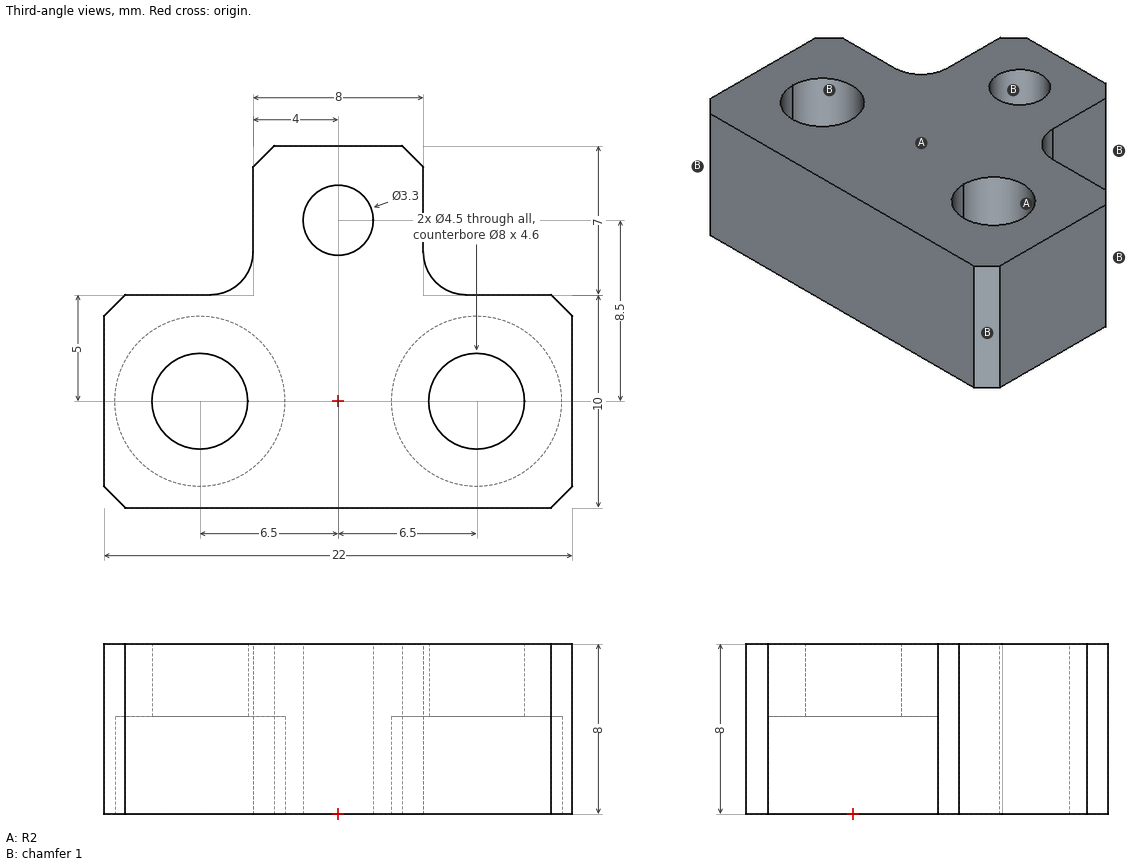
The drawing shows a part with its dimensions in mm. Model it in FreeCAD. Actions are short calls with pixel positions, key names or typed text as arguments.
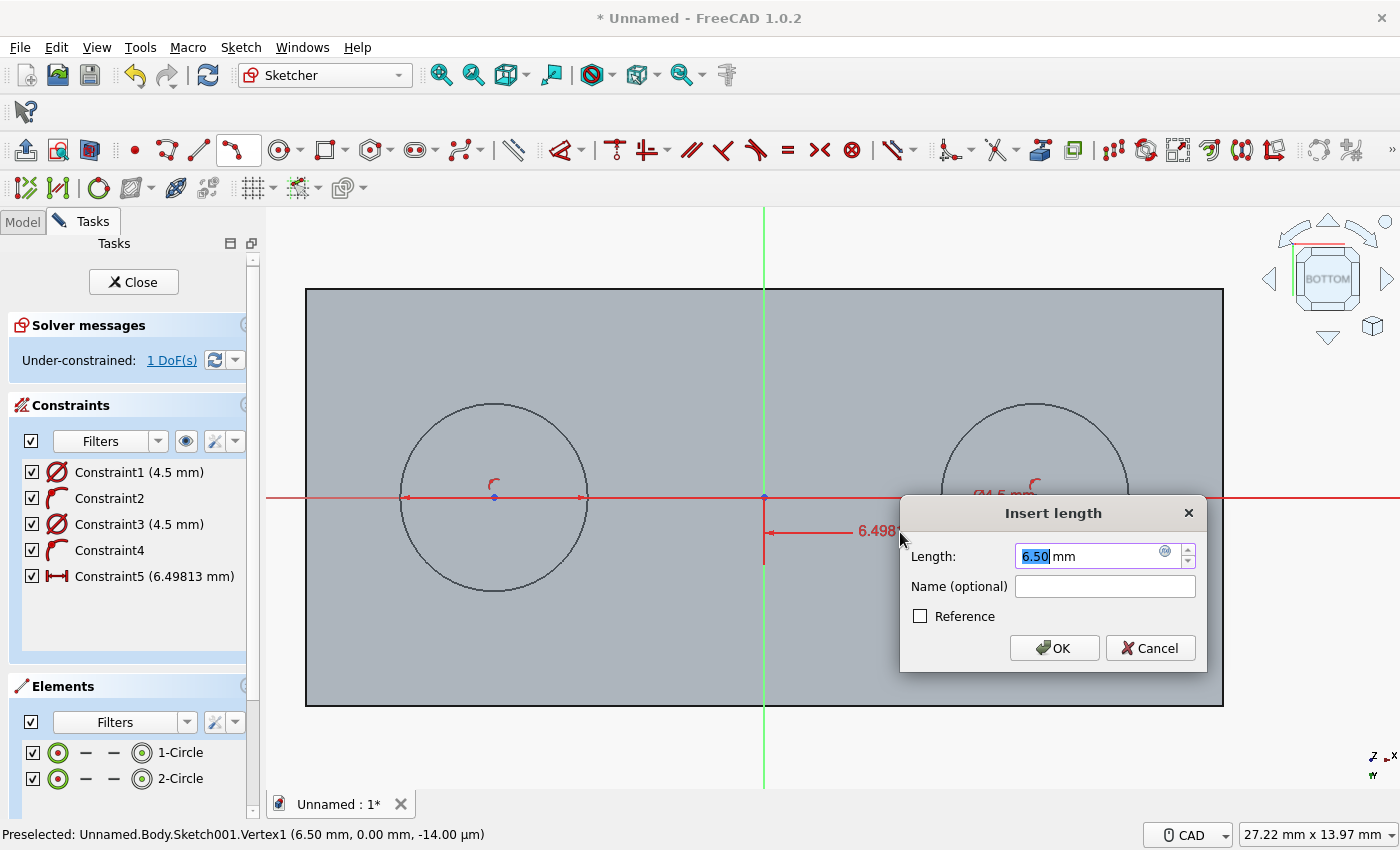
text(6.5)
key(Return)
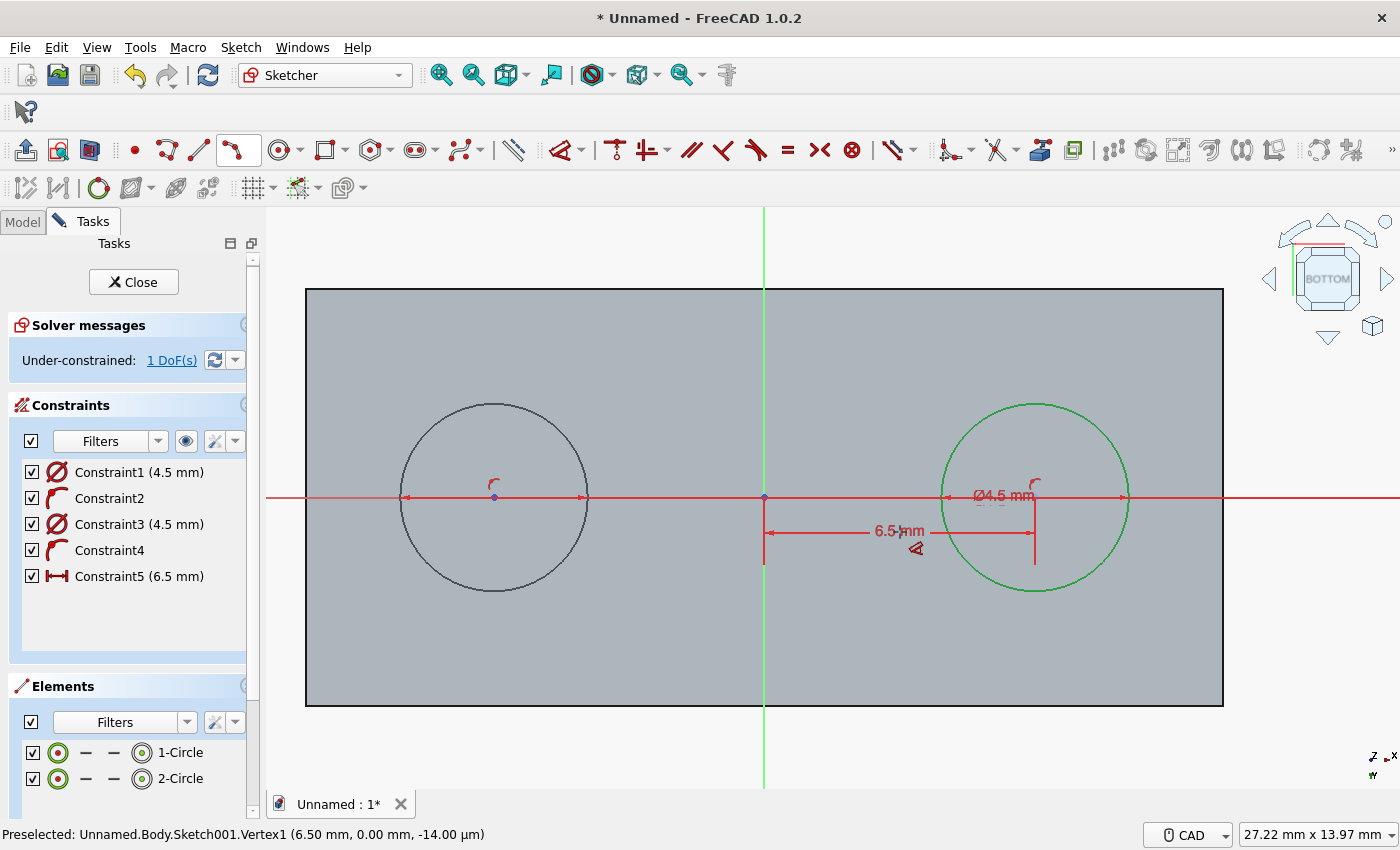
click(494, 498)
click(629, 532)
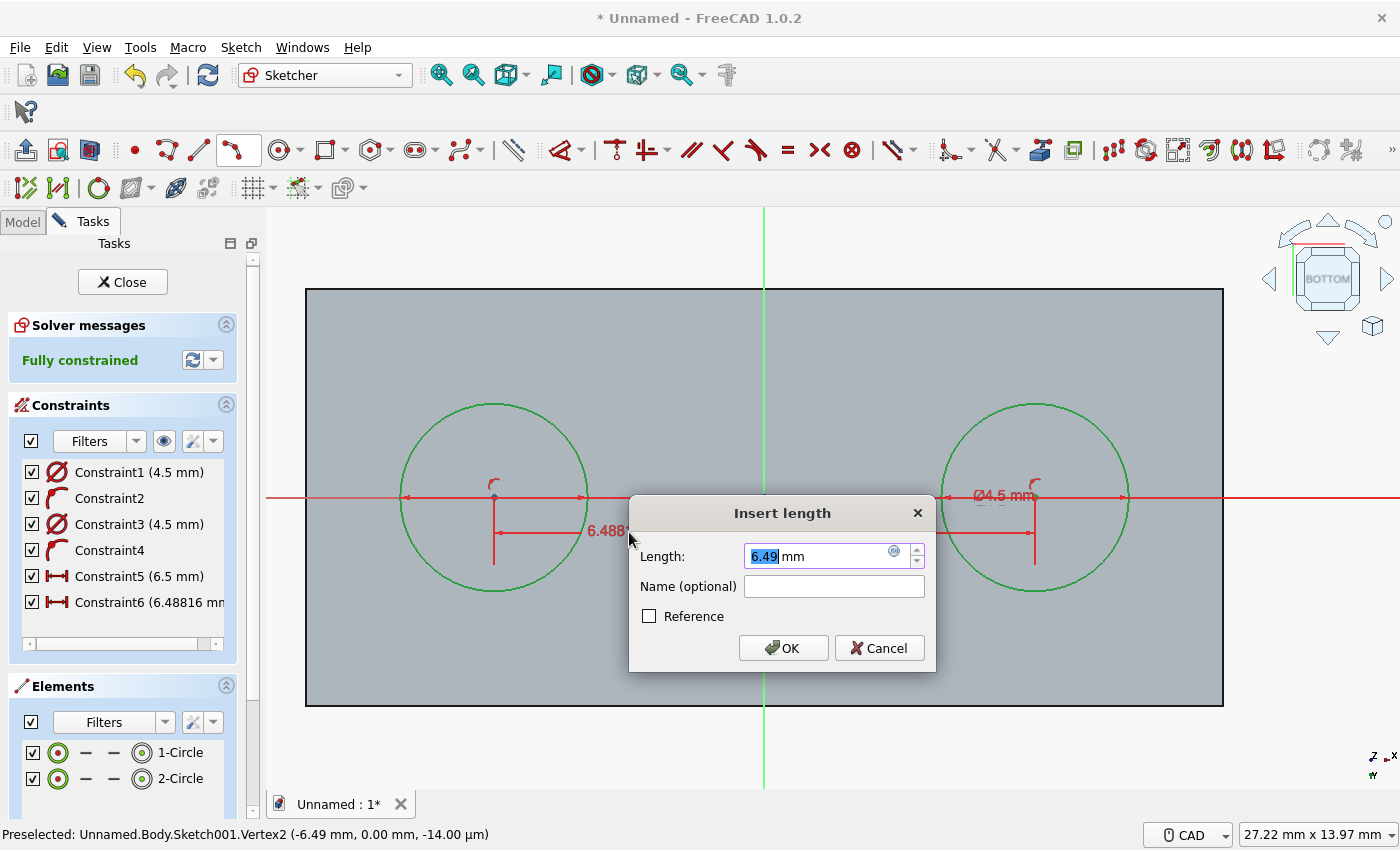
text(6.5)
key(Return)
key(Escape)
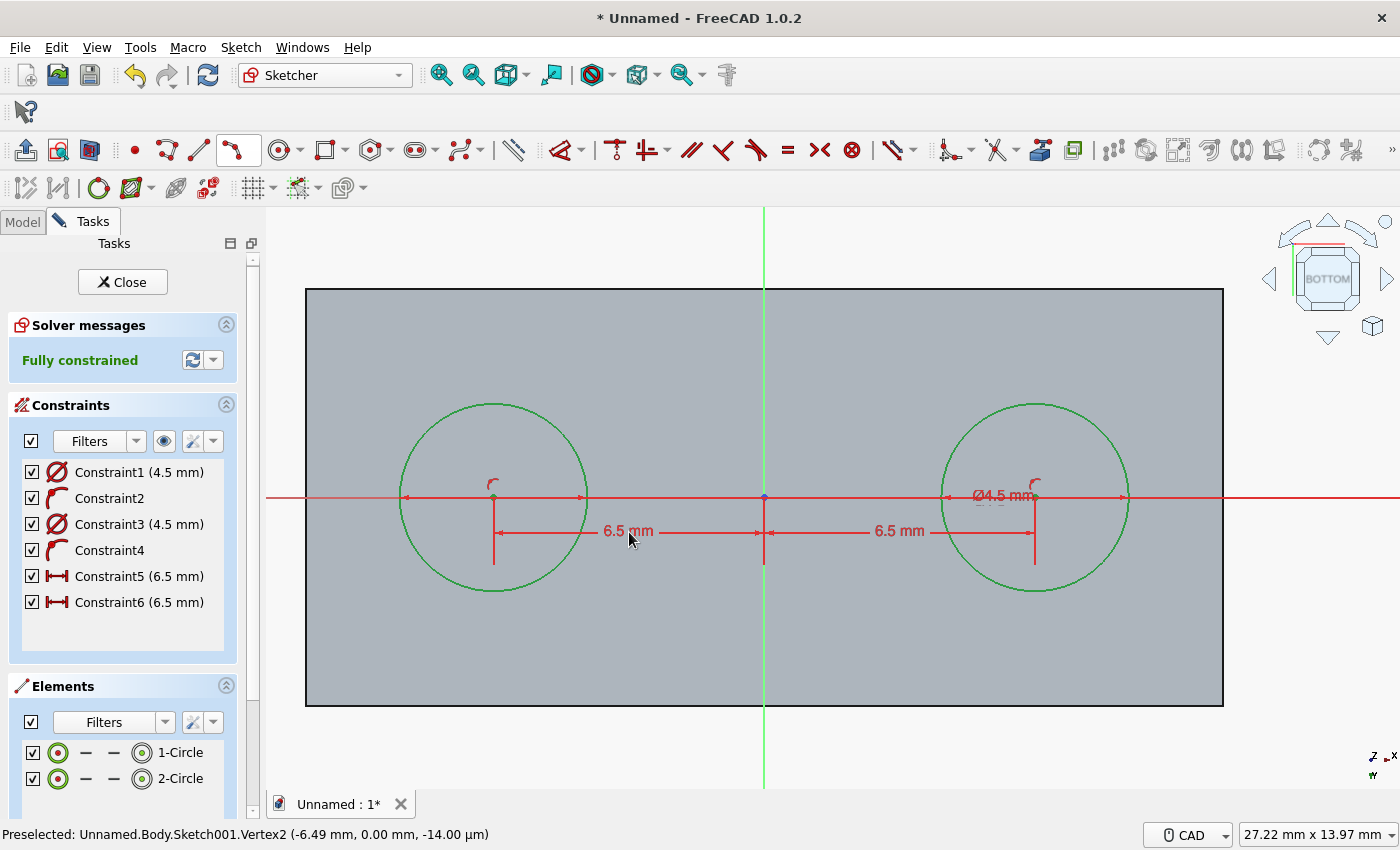
click(123, 282)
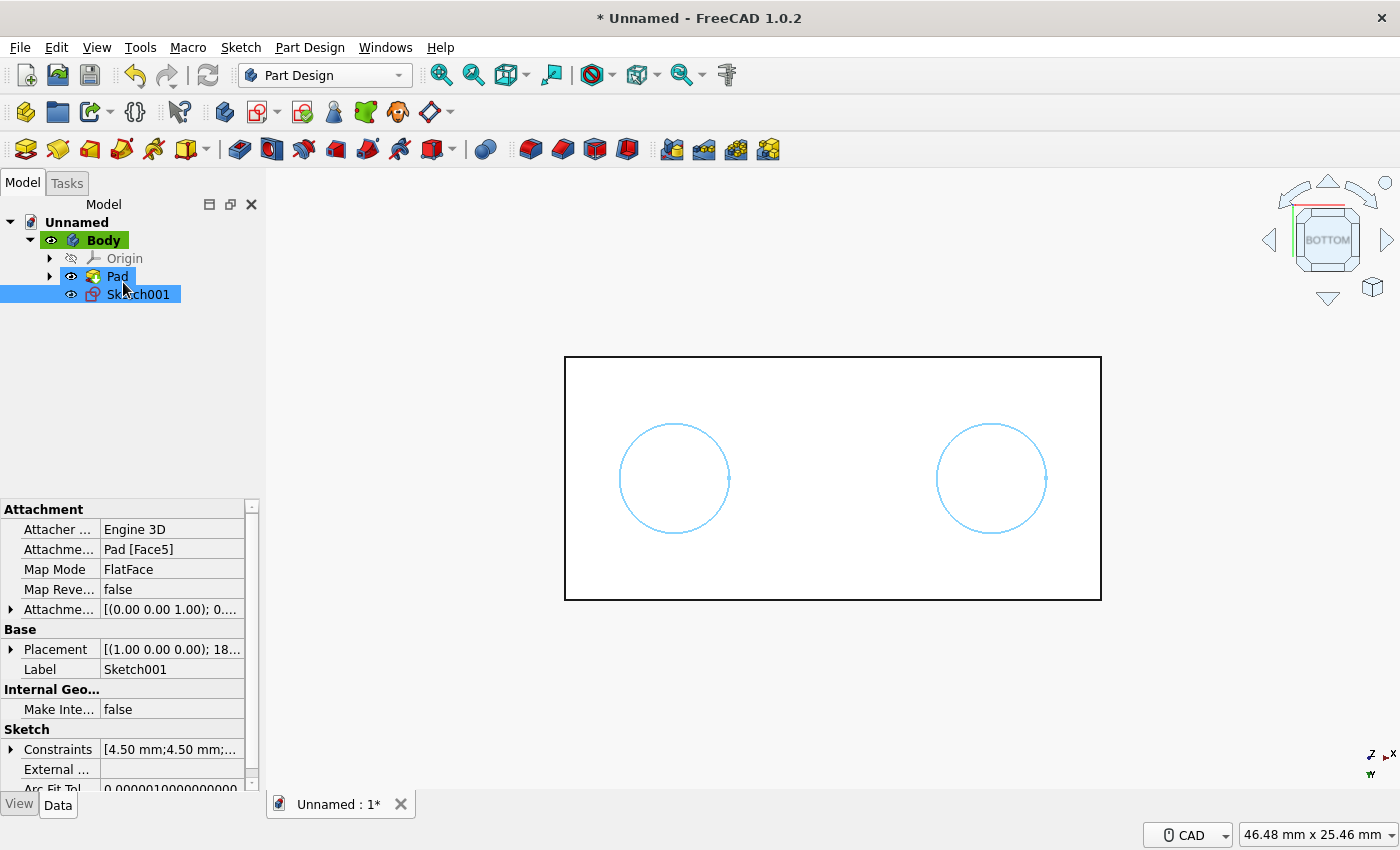
click(272, 150)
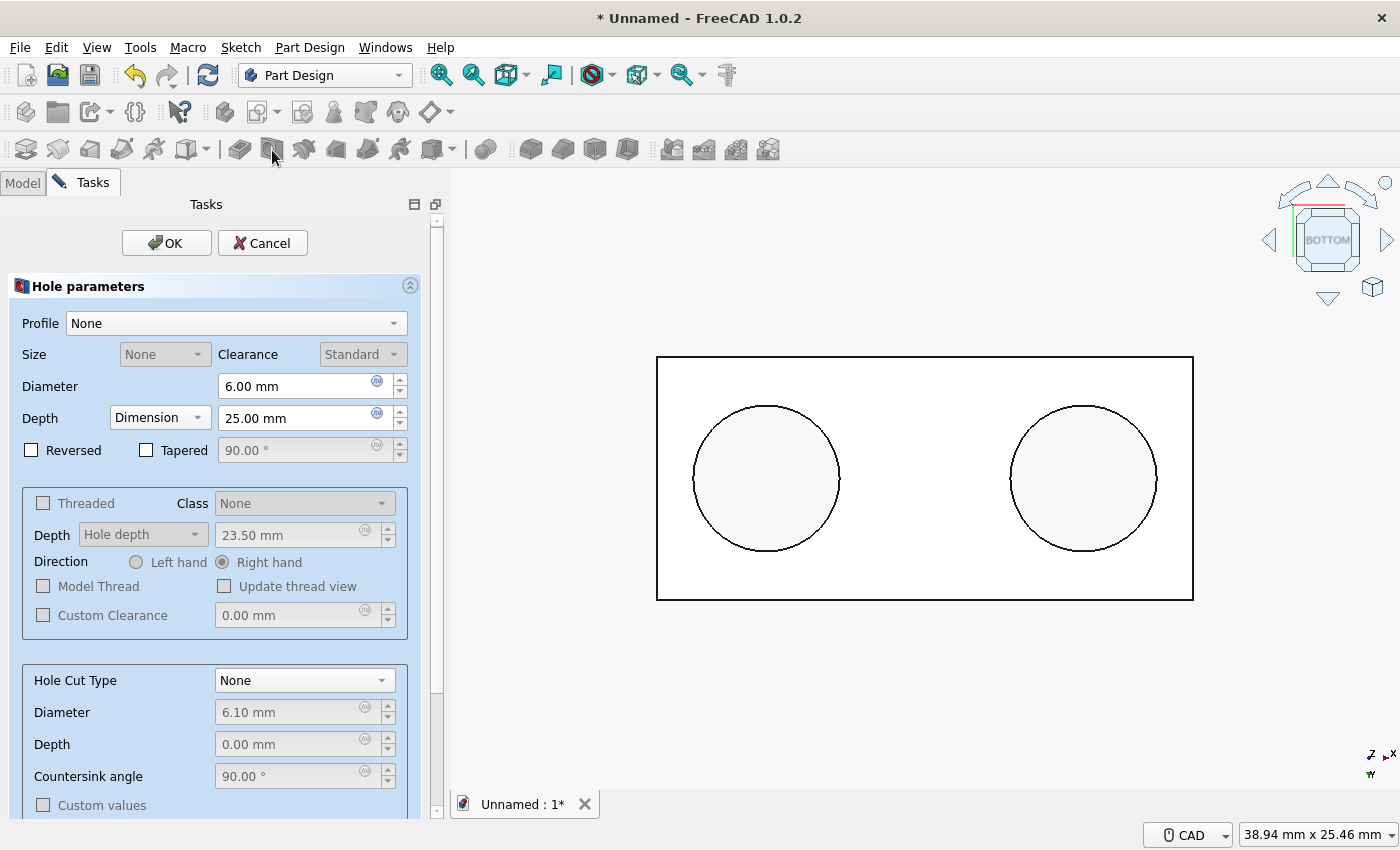
triple_click(305, 386)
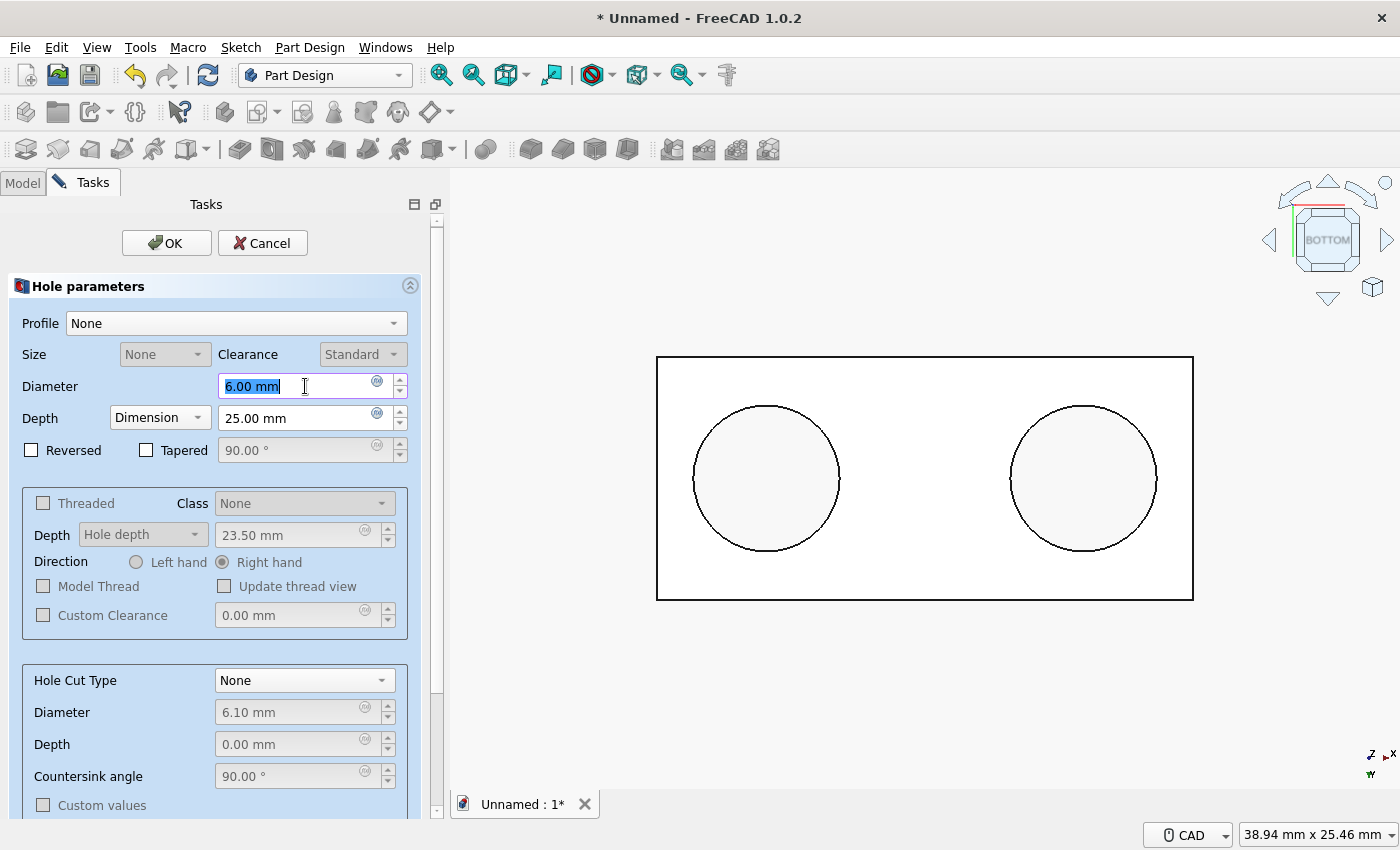
text(4.5)
key(Tab)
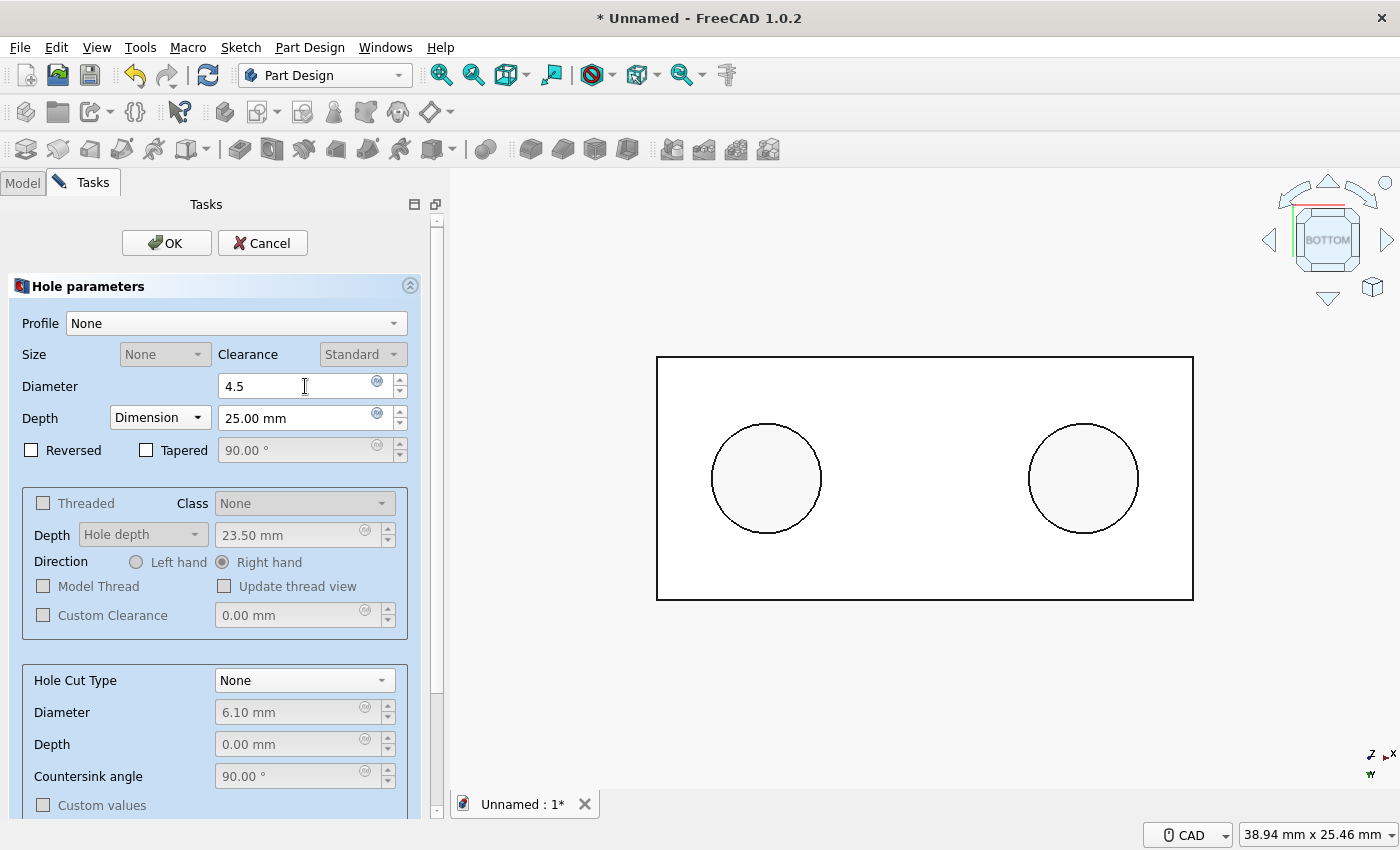
click(161, 418)